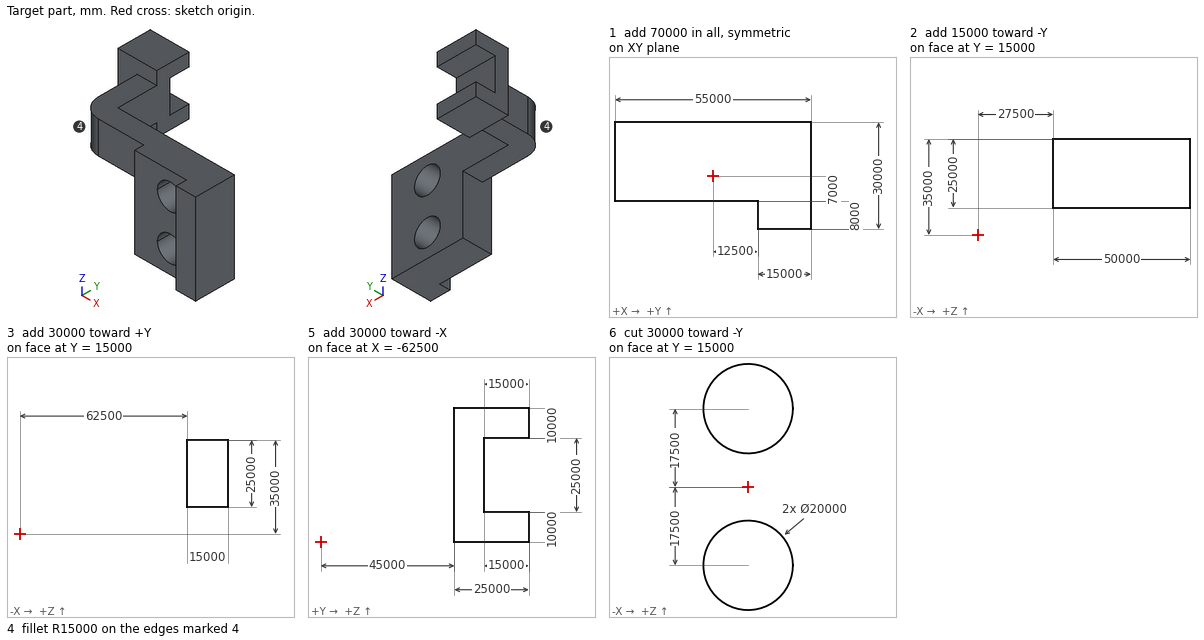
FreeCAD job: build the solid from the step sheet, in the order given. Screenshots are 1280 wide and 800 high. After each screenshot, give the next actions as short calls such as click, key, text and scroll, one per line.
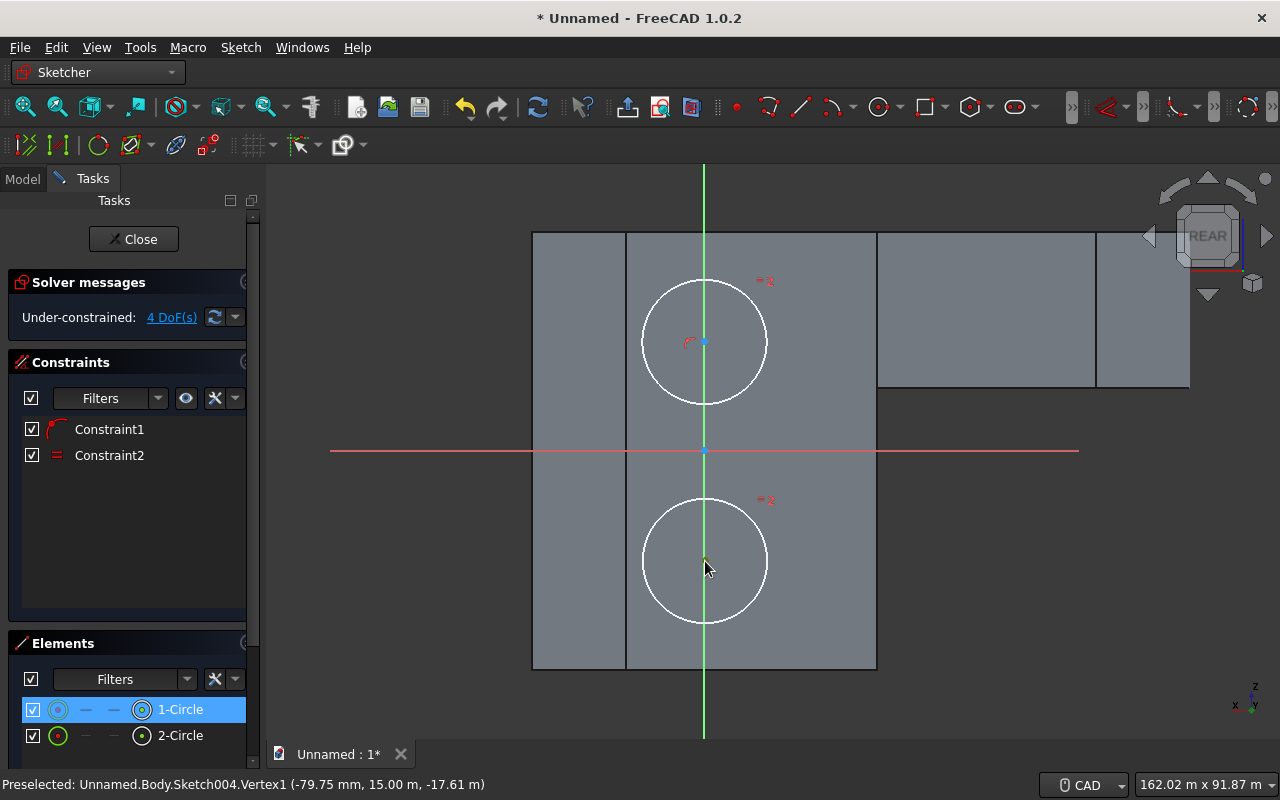
click(705, 674)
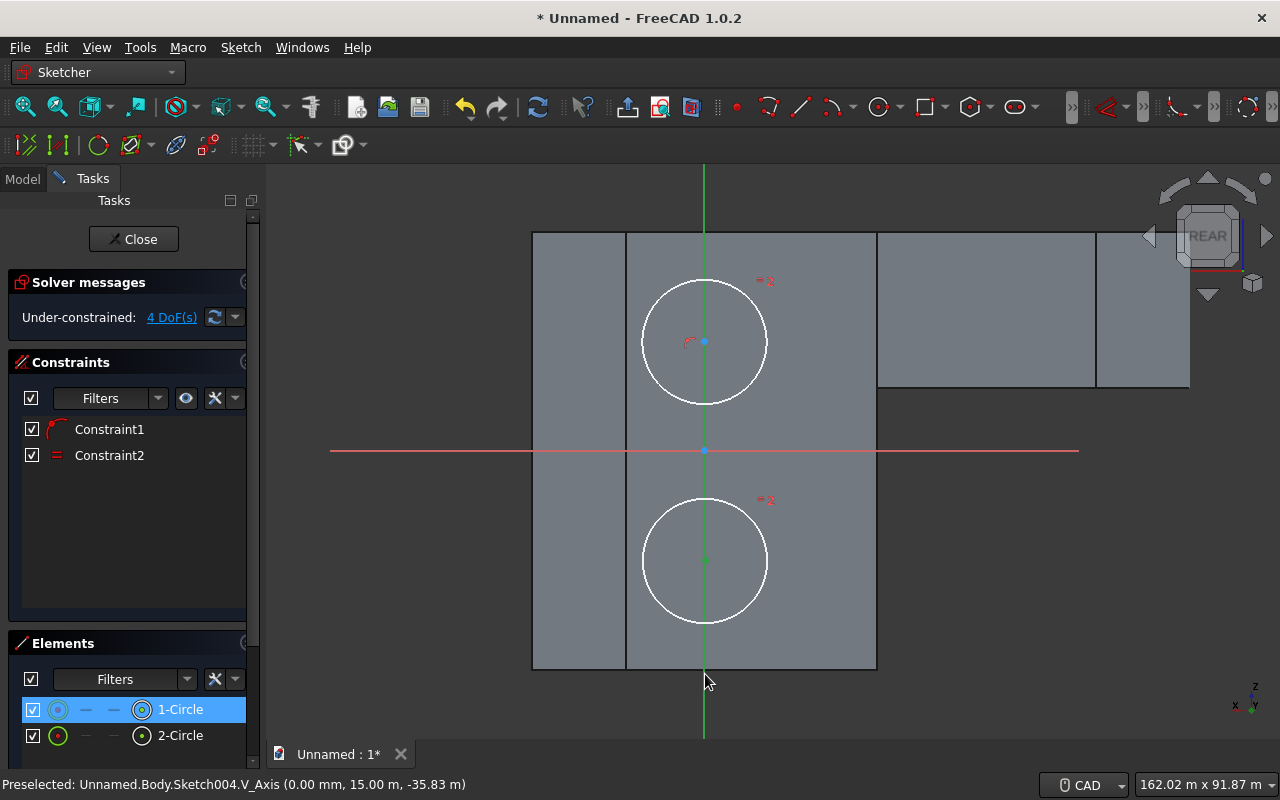
key(c)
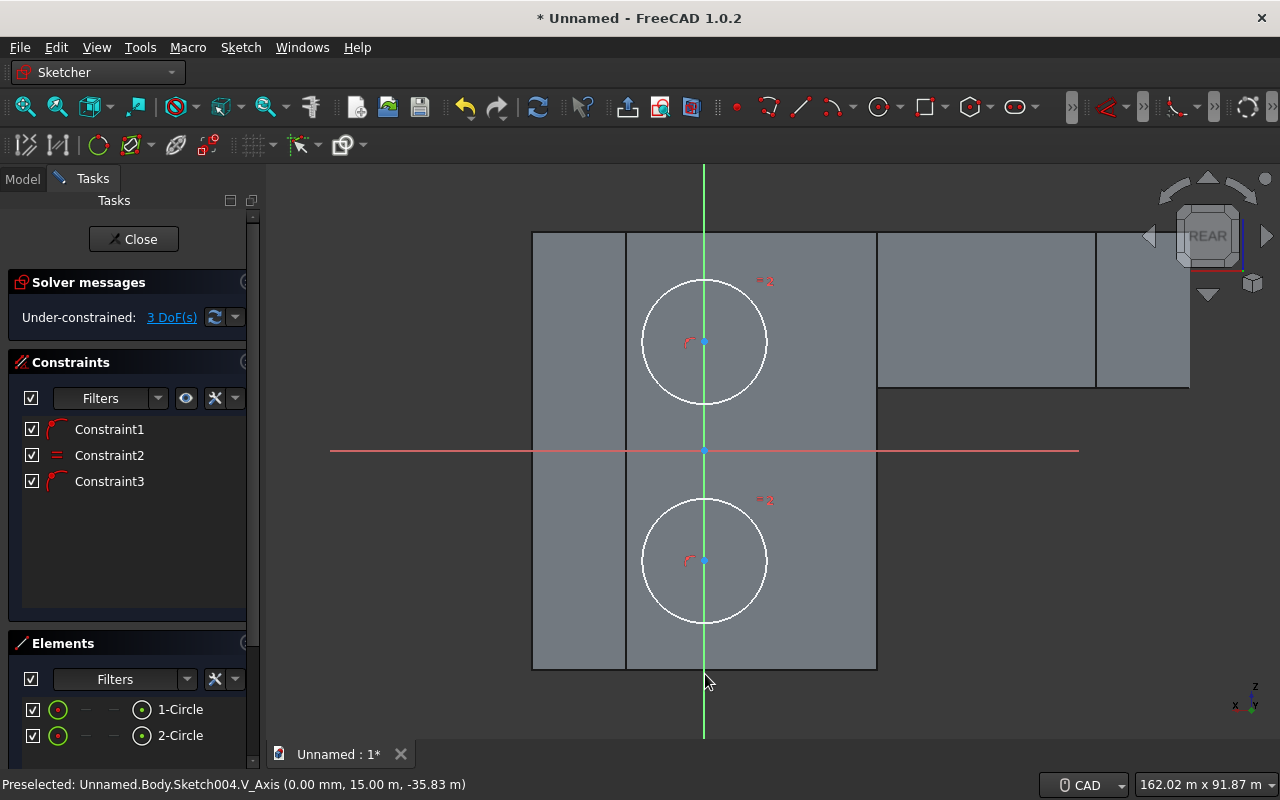
key(d)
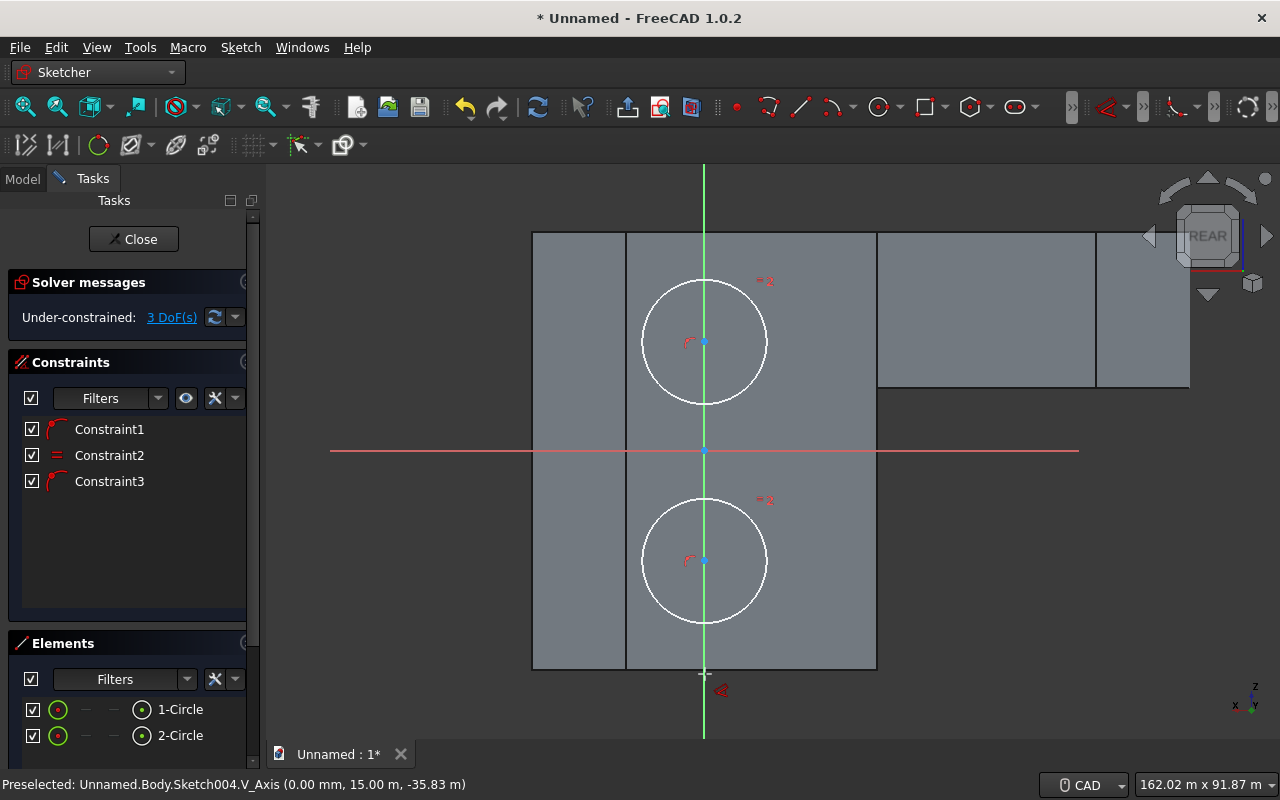
click(748, 517)
click(770, 494)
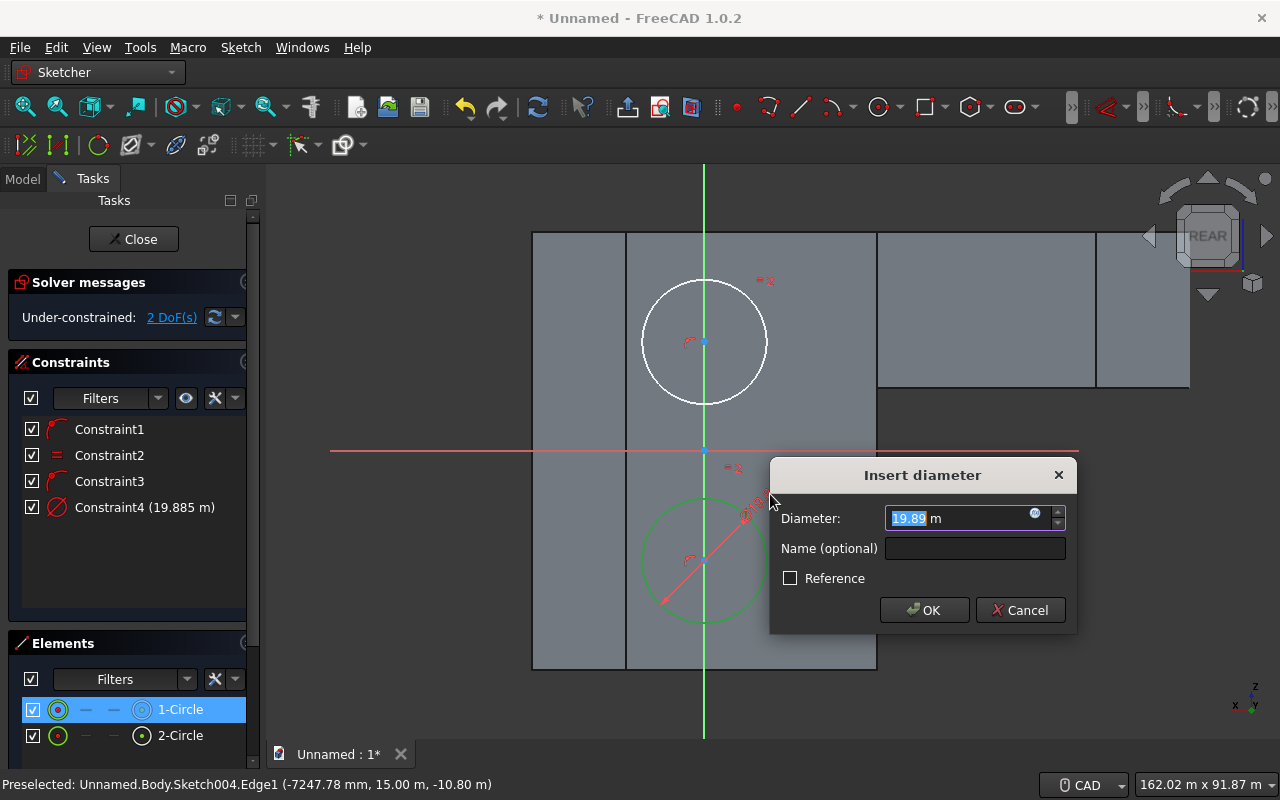
key(ctrl+a)
text(20000 mm)
key(Return)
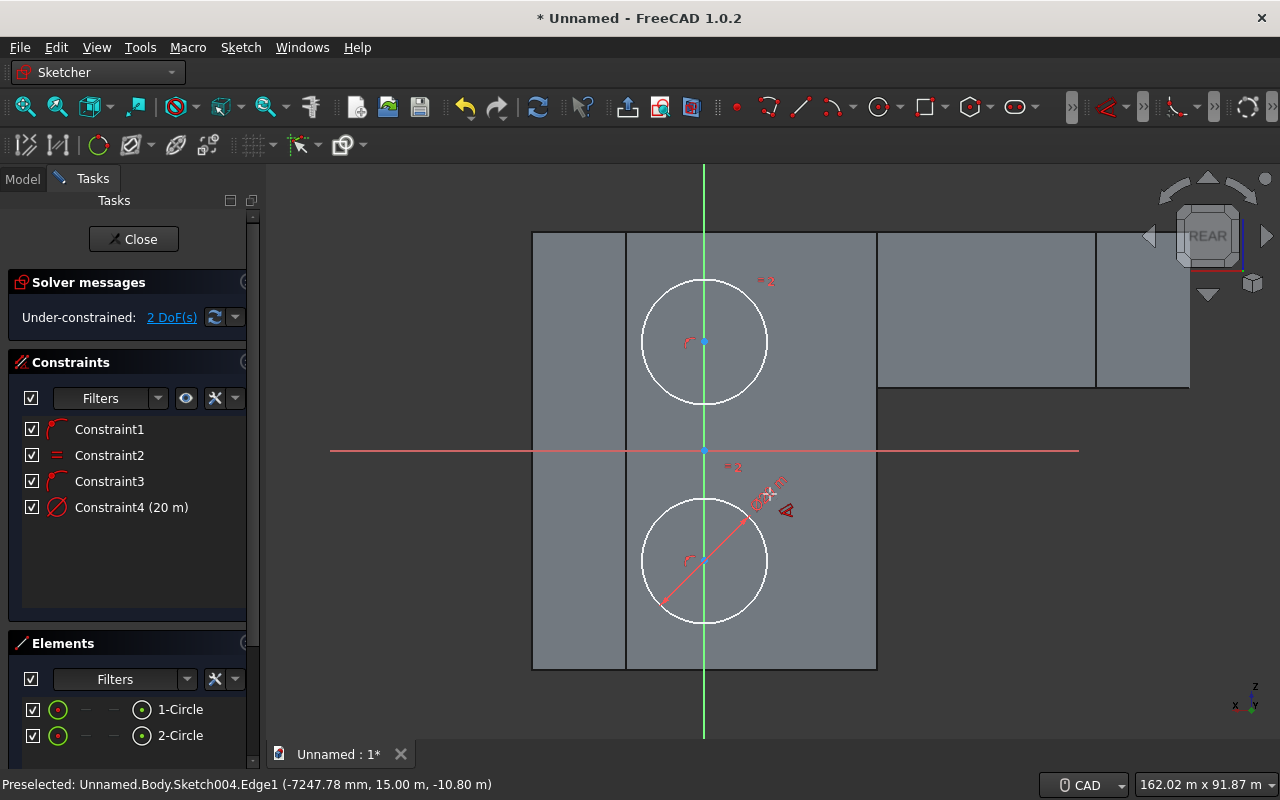
click(705, 561)
click(739, 531)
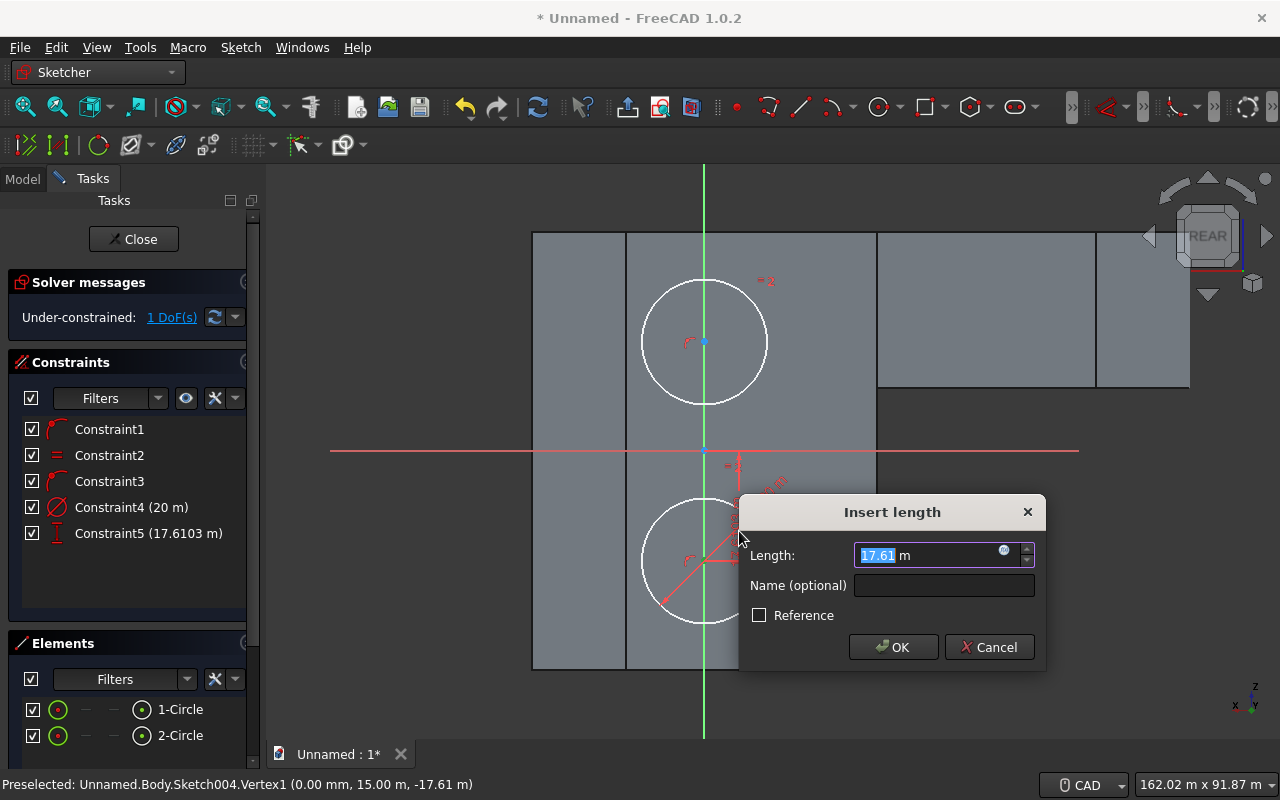
key(ctrl+a)
text(17500 mm)
key(Return)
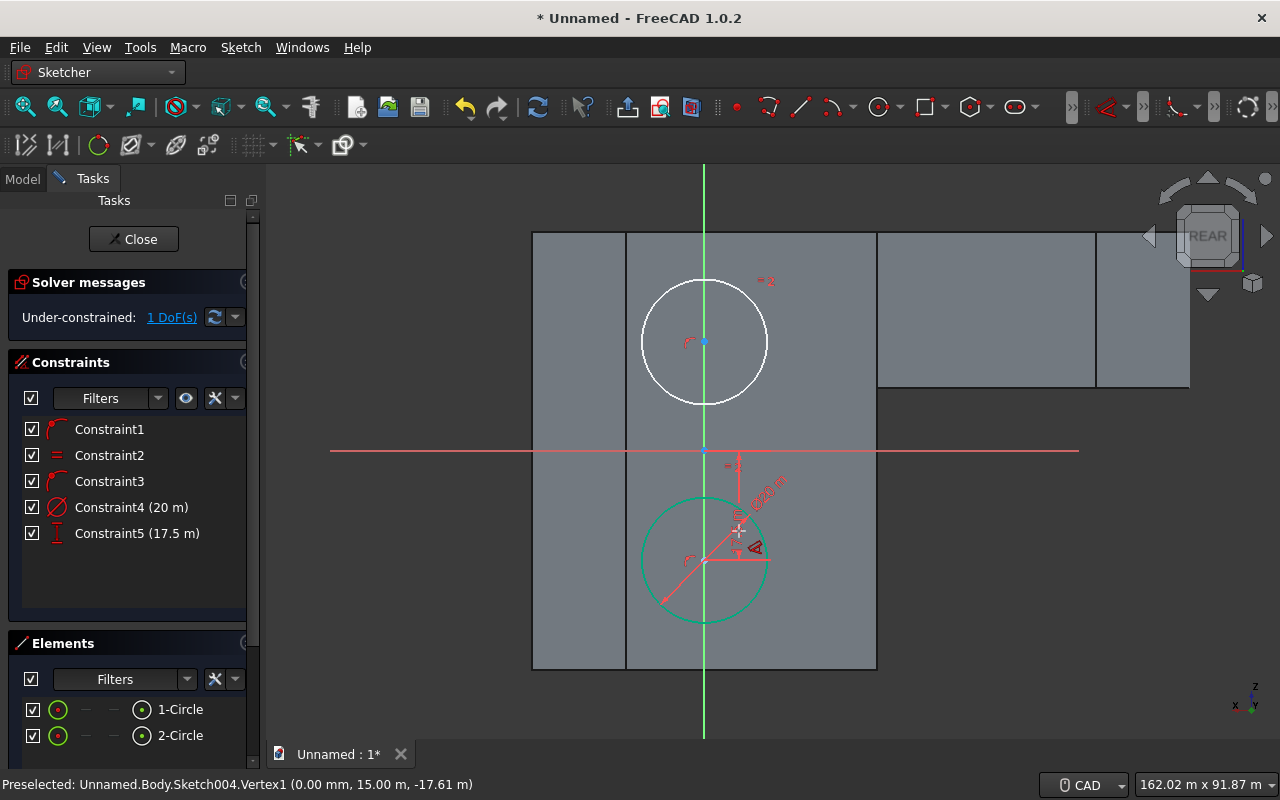
click(705, 342)
click(739, 371)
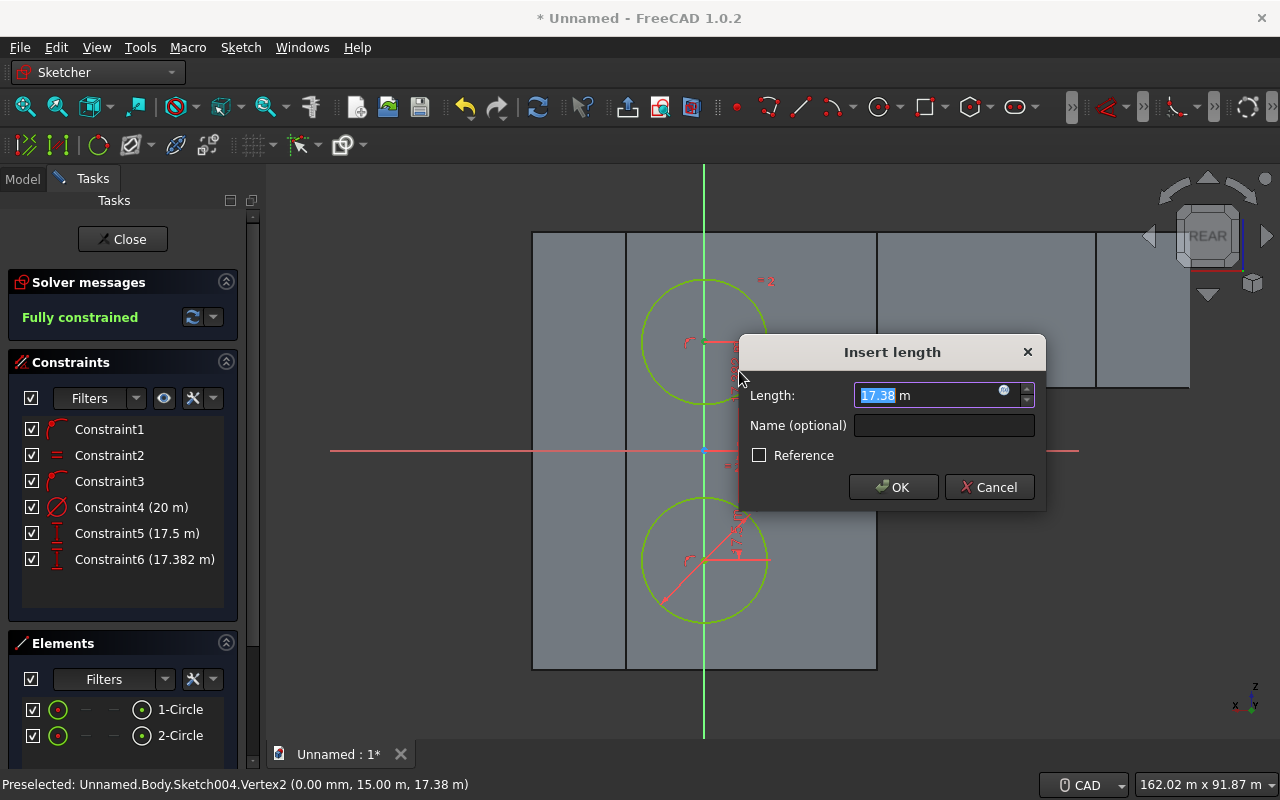
key(ctrl+a)
text(17500 mm)
key(Return)
key(Escape)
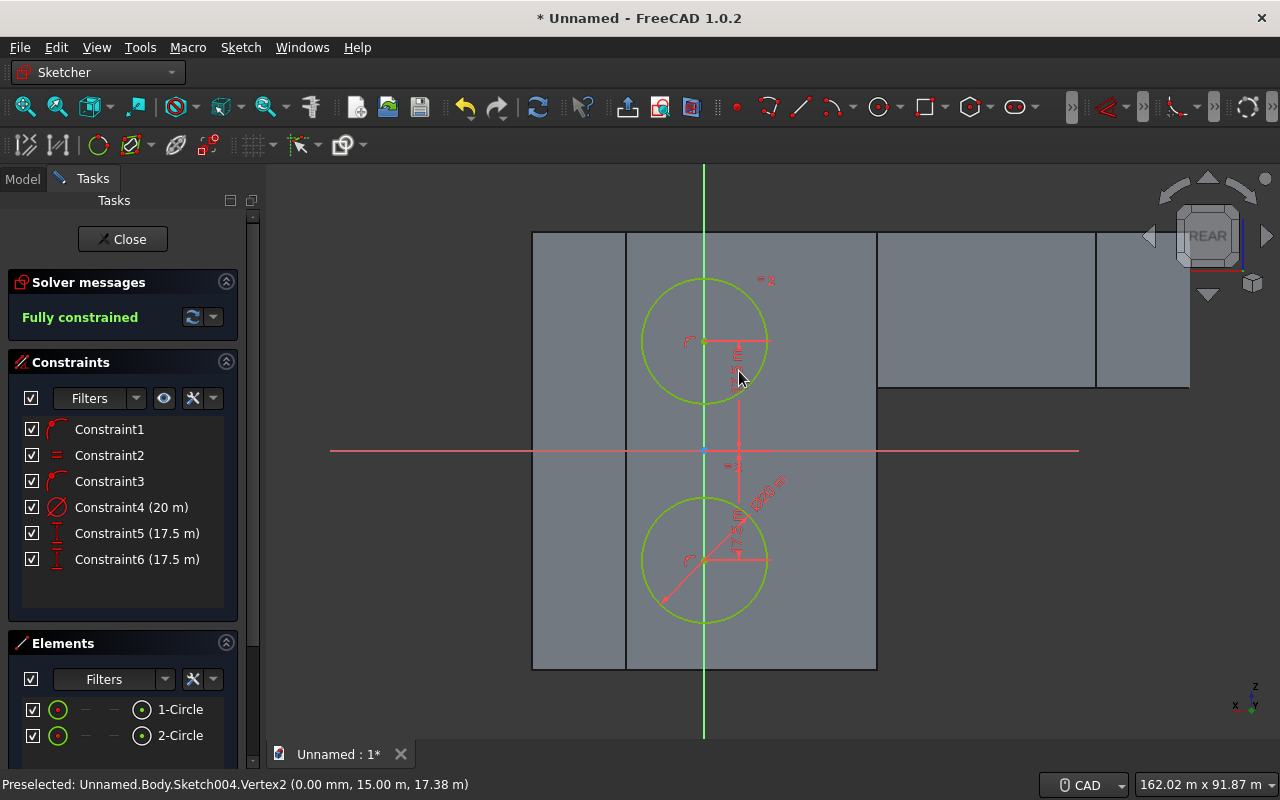
click(123, 239)